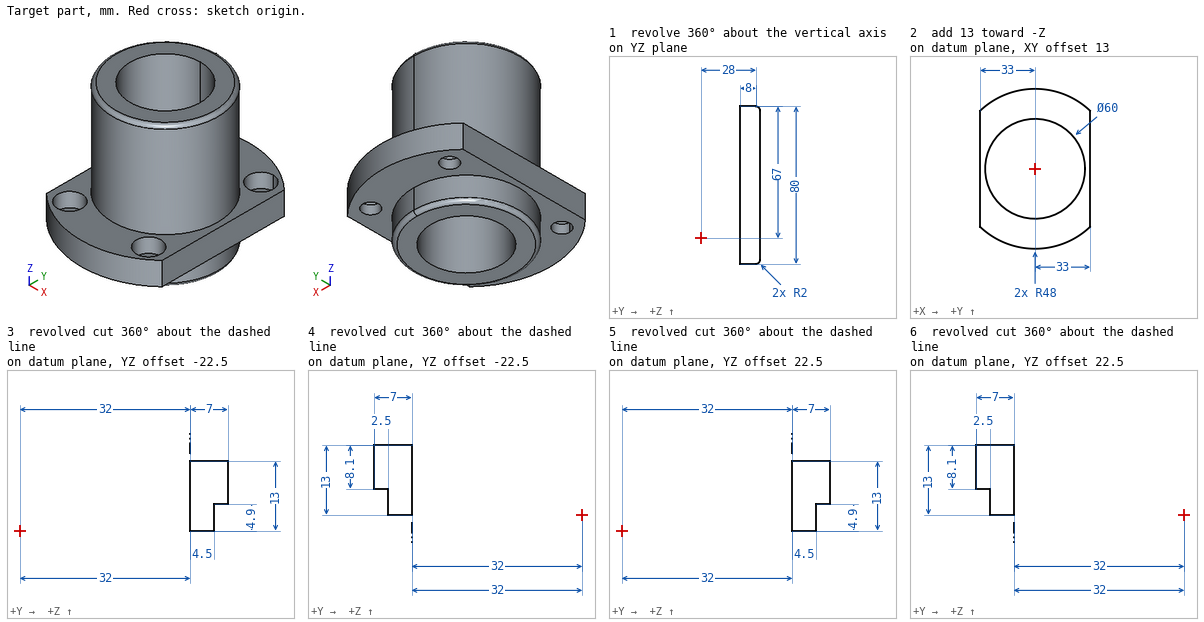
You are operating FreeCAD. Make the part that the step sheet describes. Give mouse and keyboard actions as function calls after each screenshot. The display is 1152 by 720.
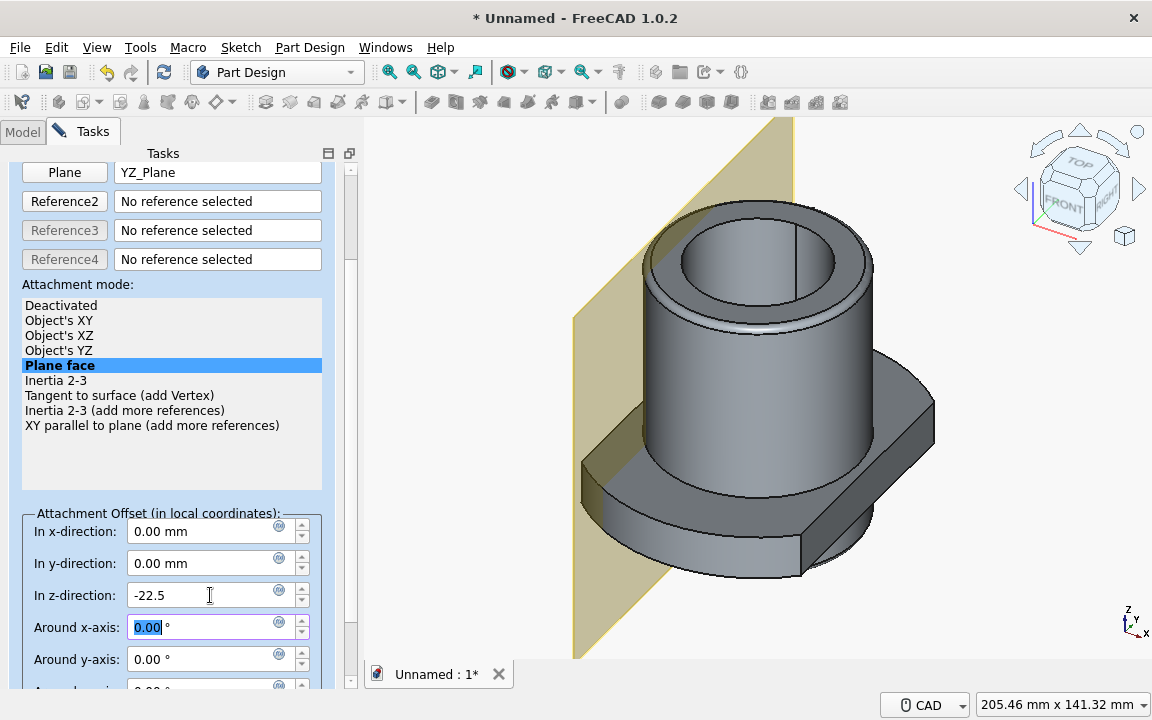
scroll(351, 426, up, 3)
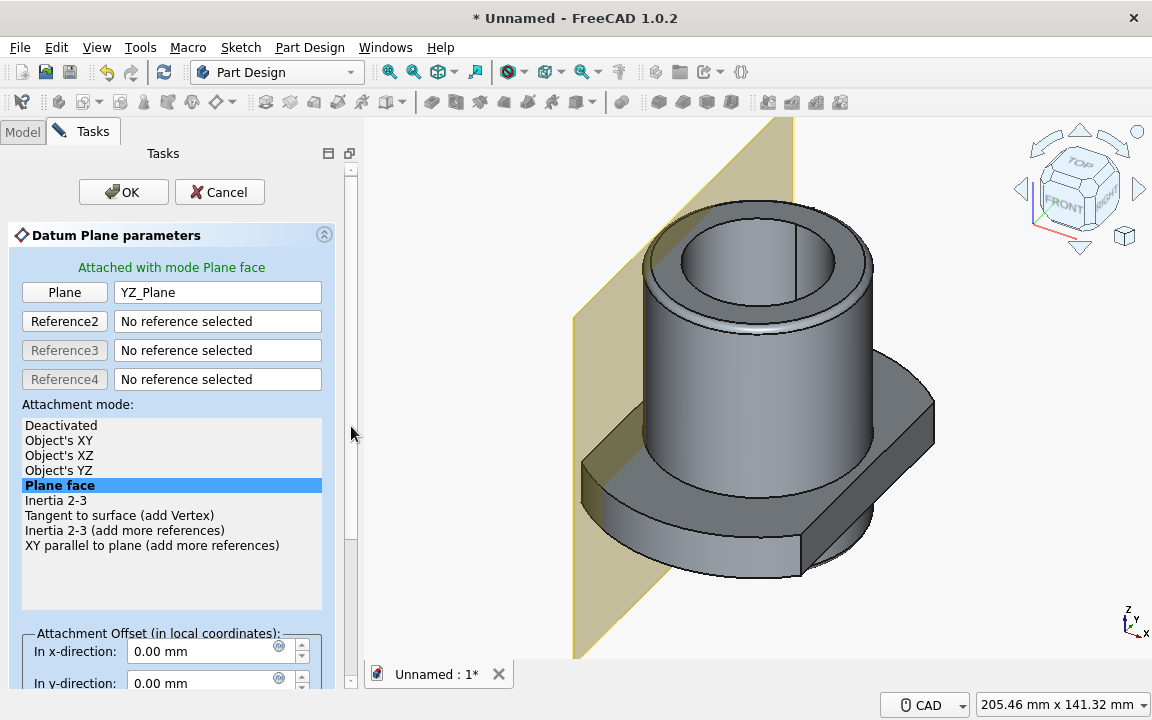
click(124, 192)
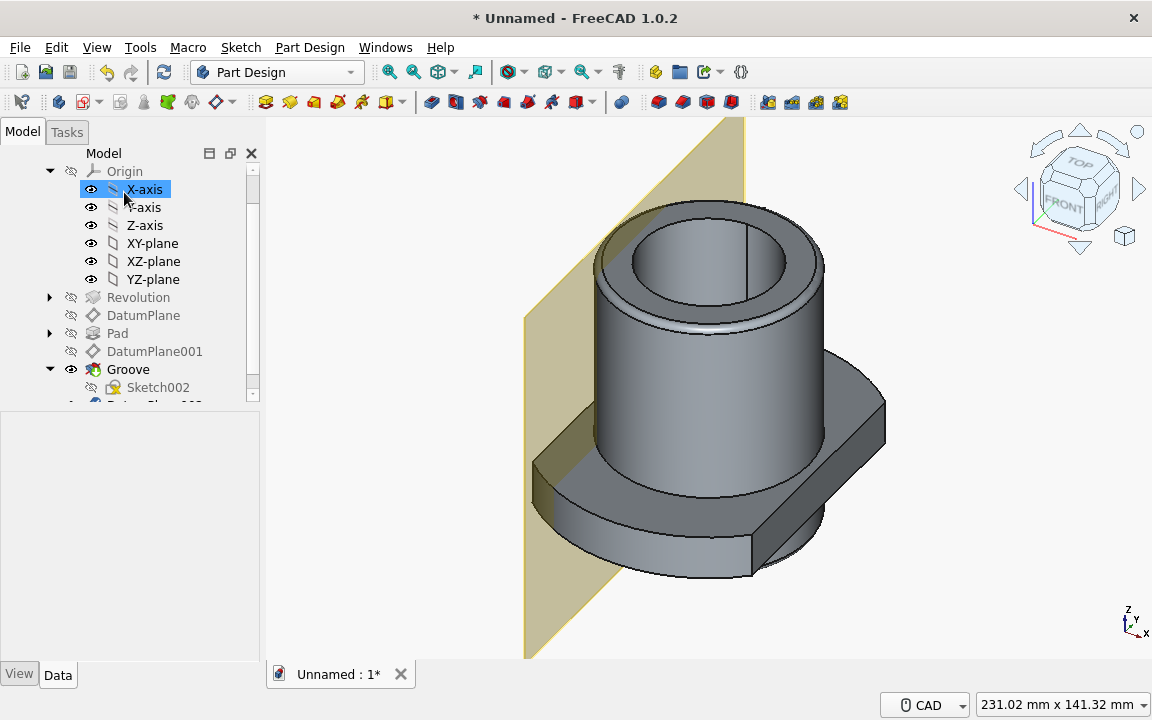
scroll(140, 275, down, 3)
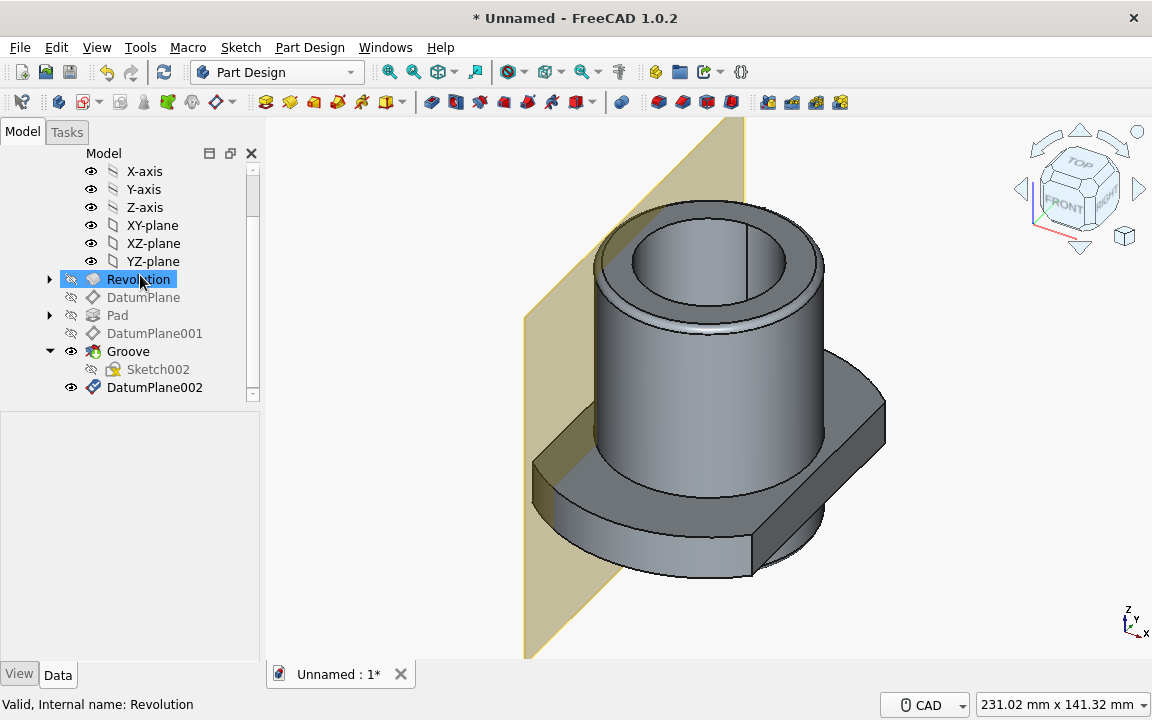
click(116, 387)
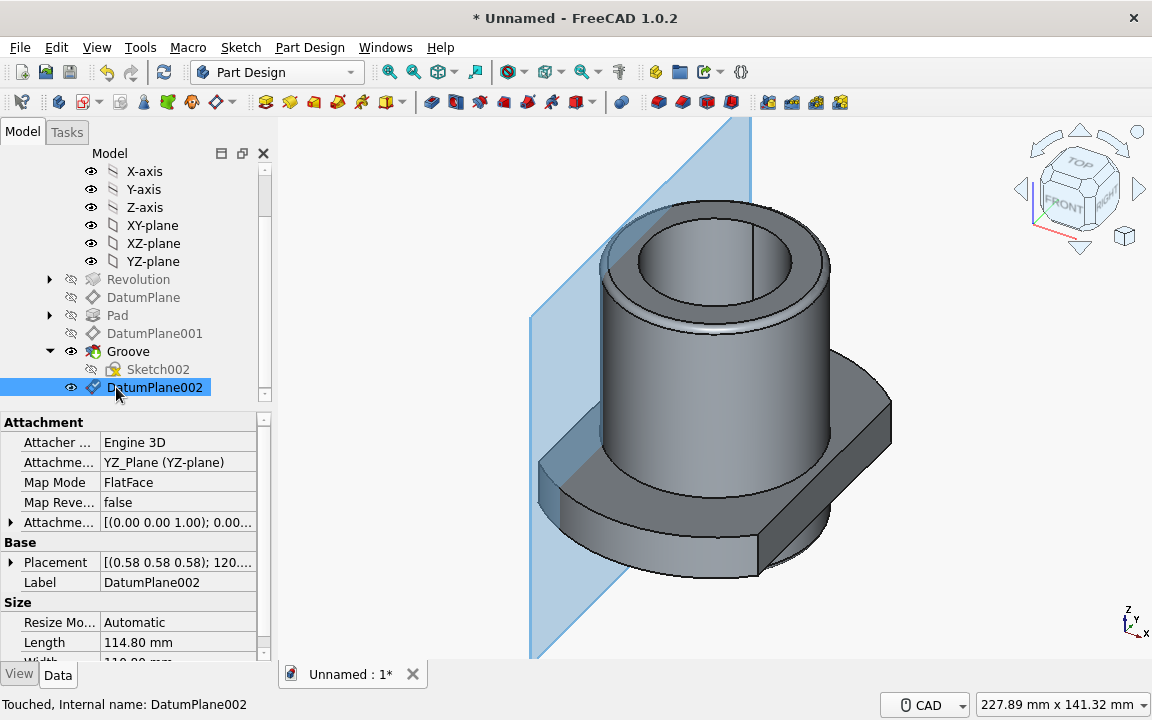
click(84, 102)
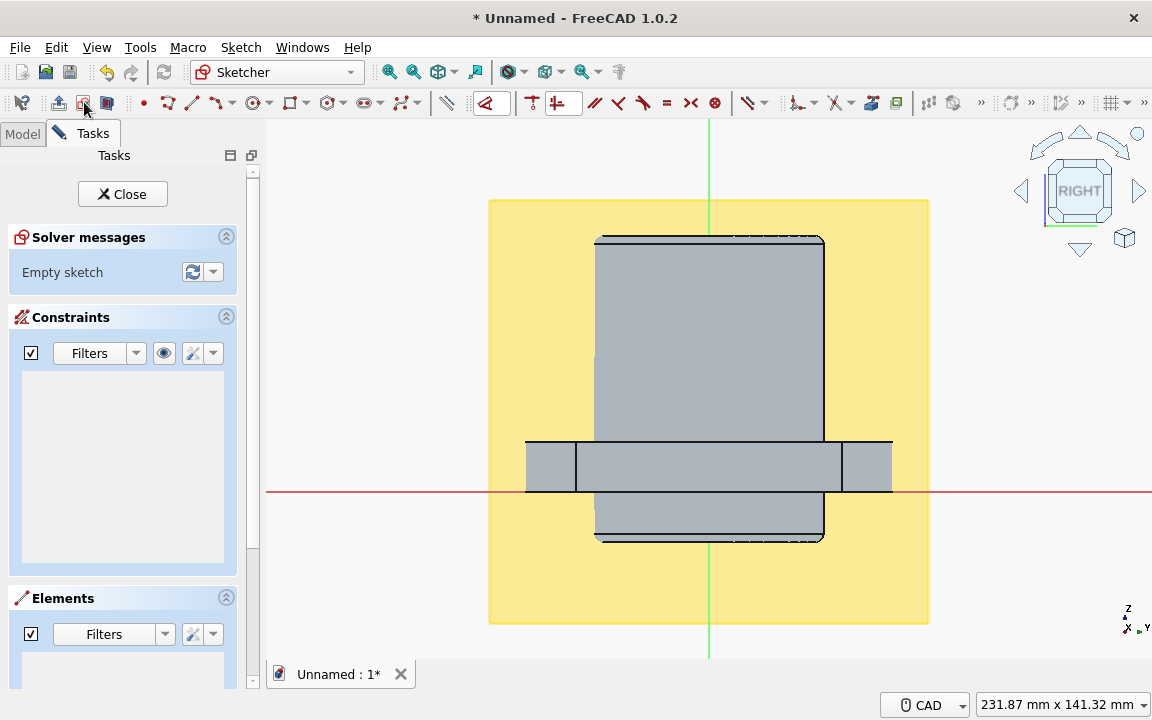
click(108, 104)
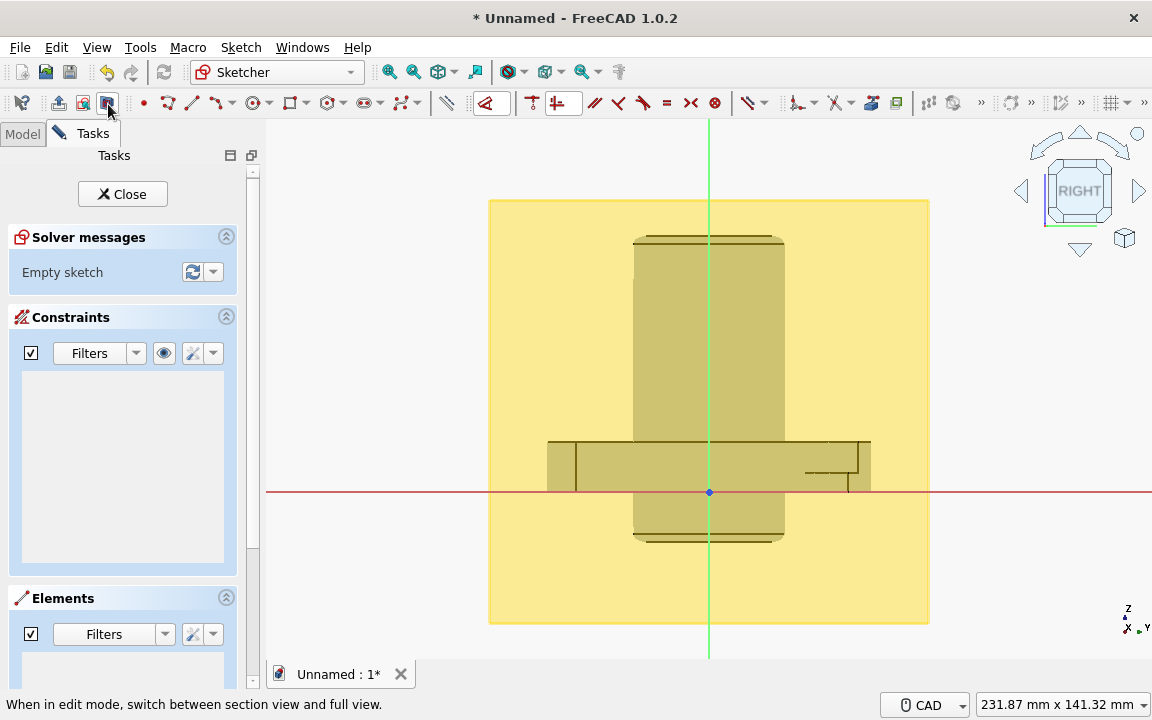
scroll(632, 515, up, 6)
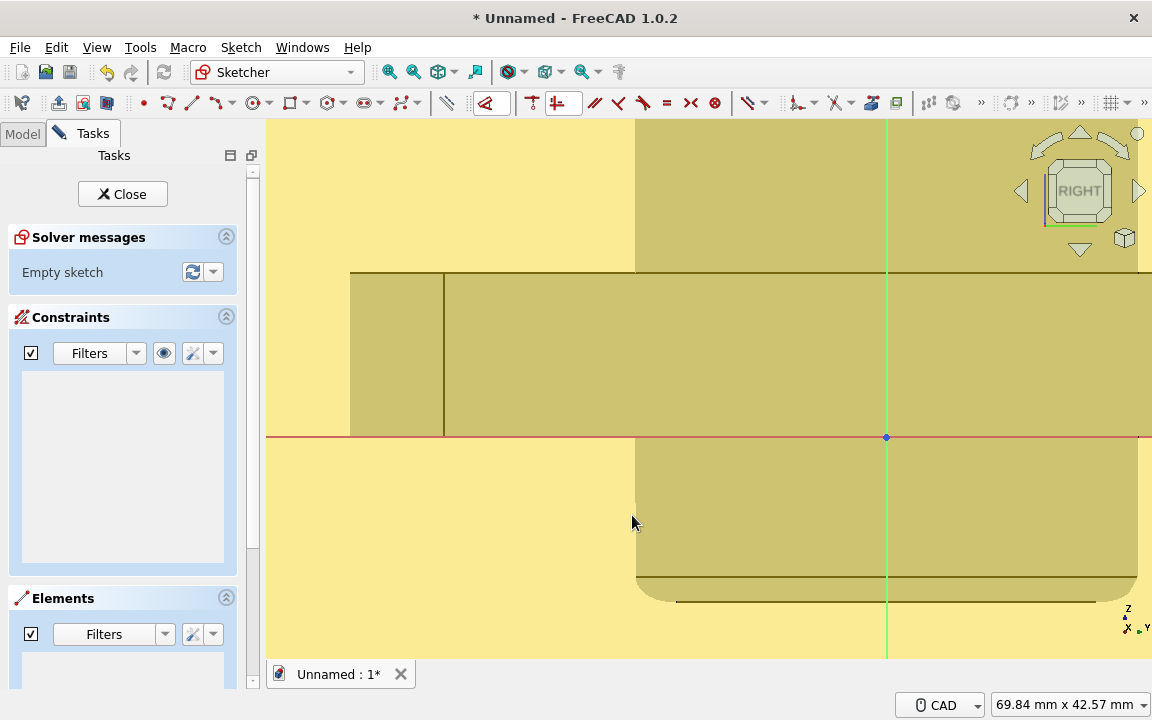
click(168, 104)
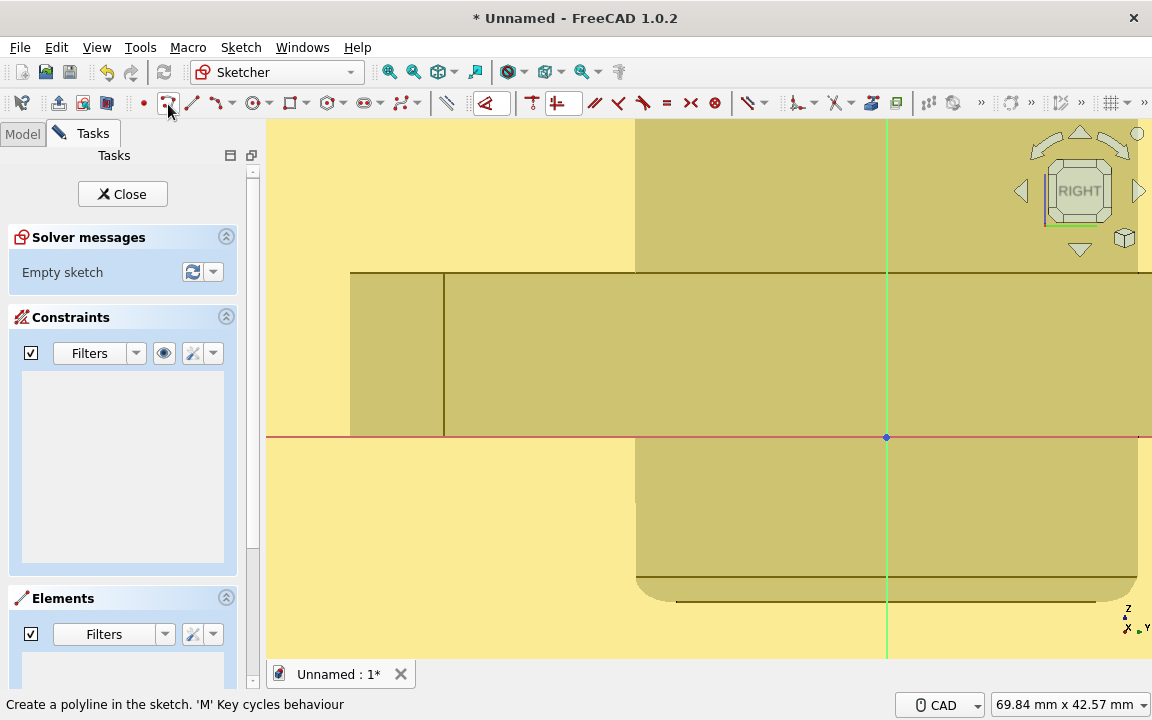
click(481, 437)
click(481, 273)
click(392, 273)
click(392, 375)
click(424, 375)
click(424, 428)
click(481, 437)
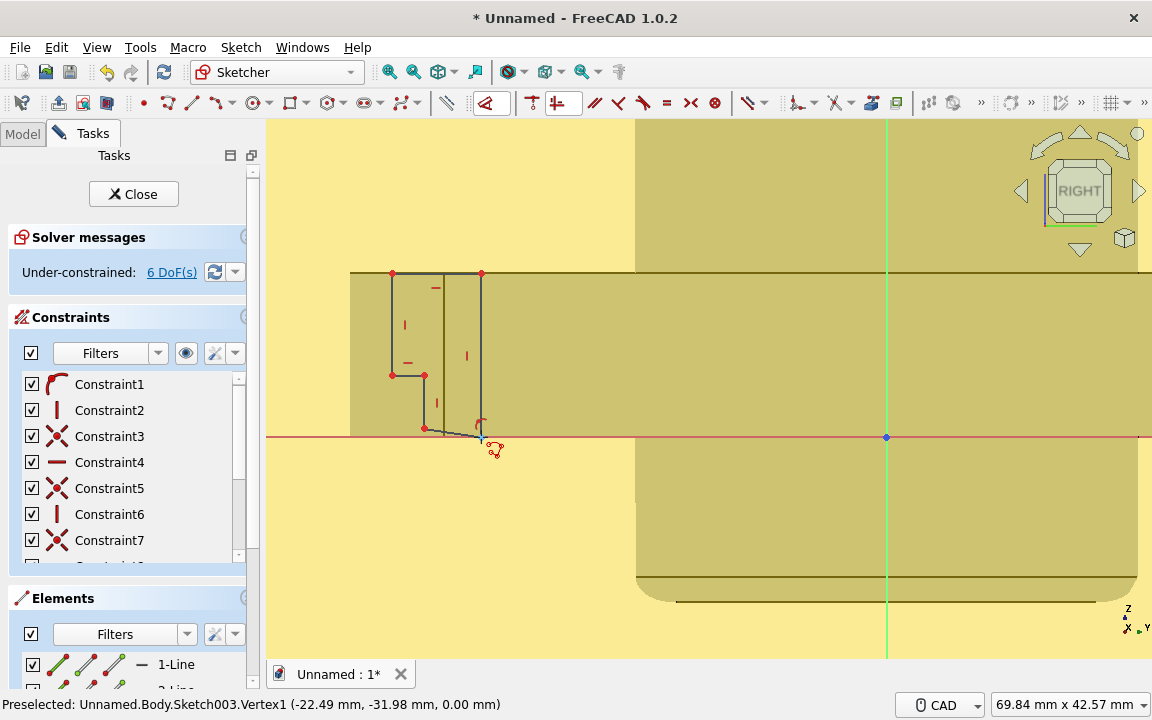
click(192, 104)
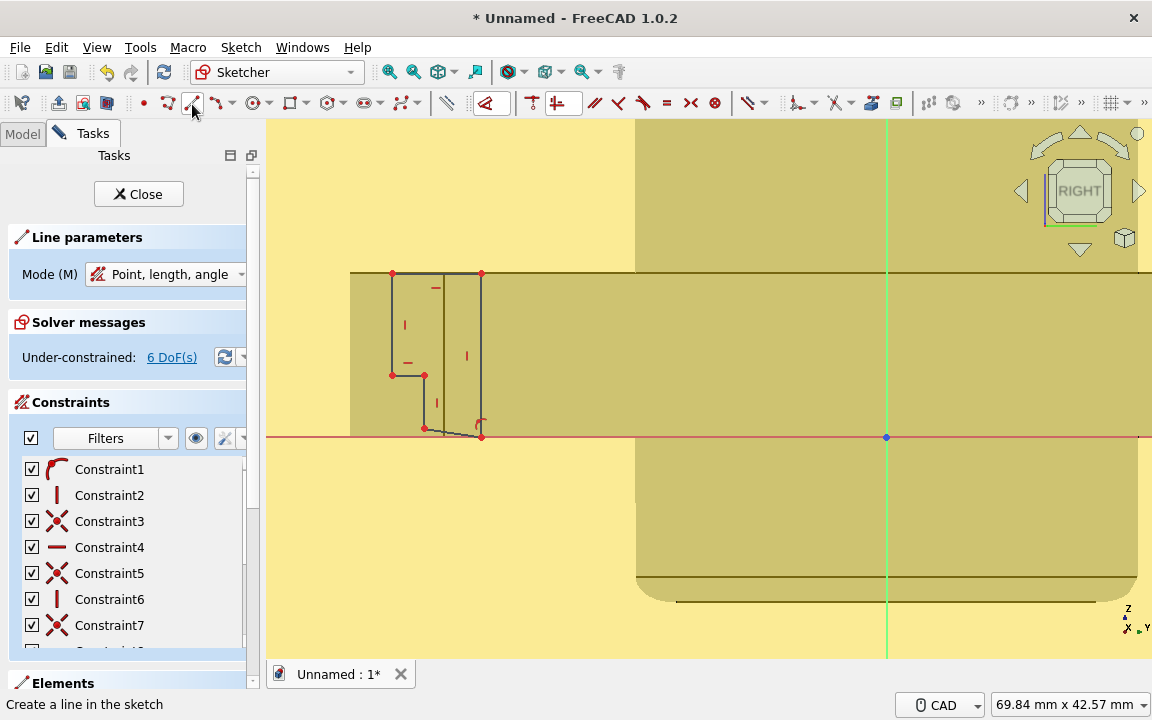
click(481, 454)
click(481, 503)
key(Escape)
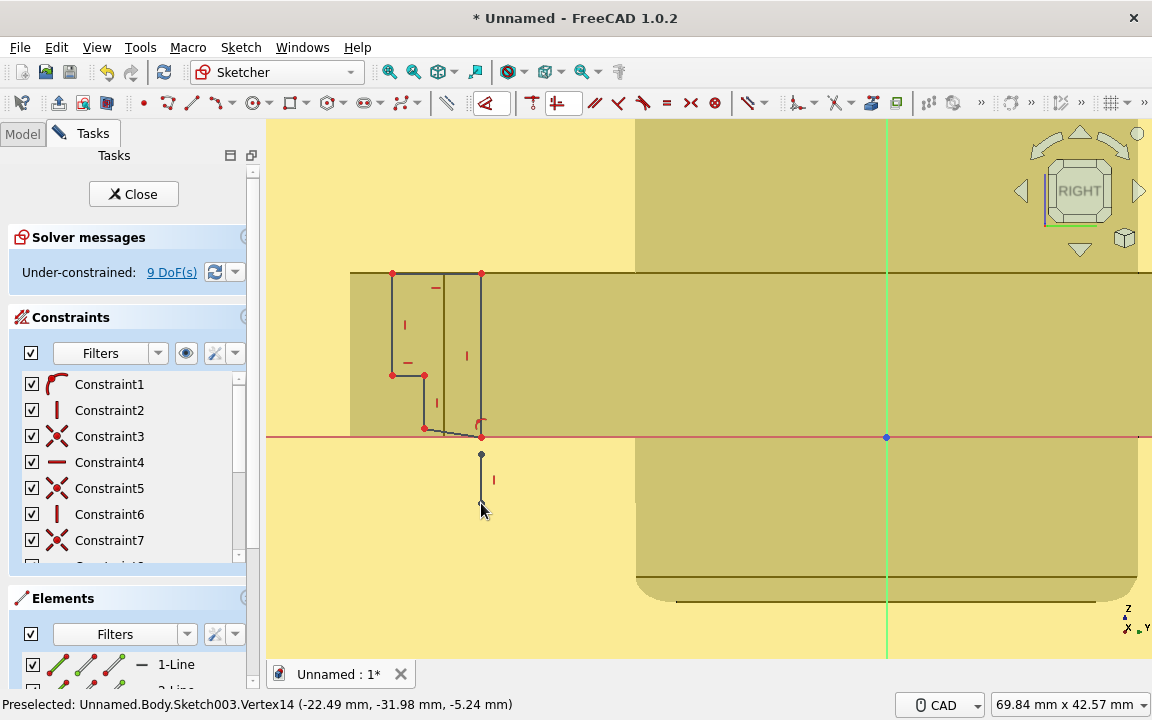
click(481, 470)